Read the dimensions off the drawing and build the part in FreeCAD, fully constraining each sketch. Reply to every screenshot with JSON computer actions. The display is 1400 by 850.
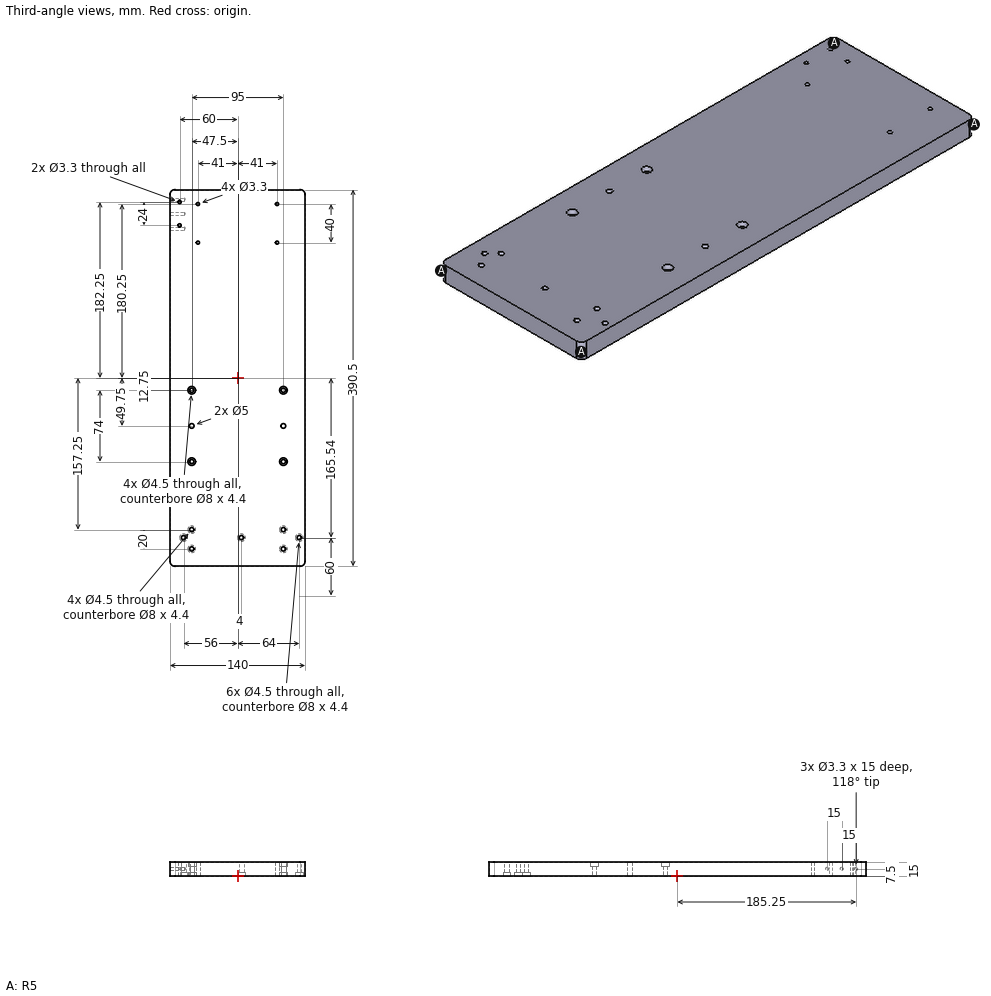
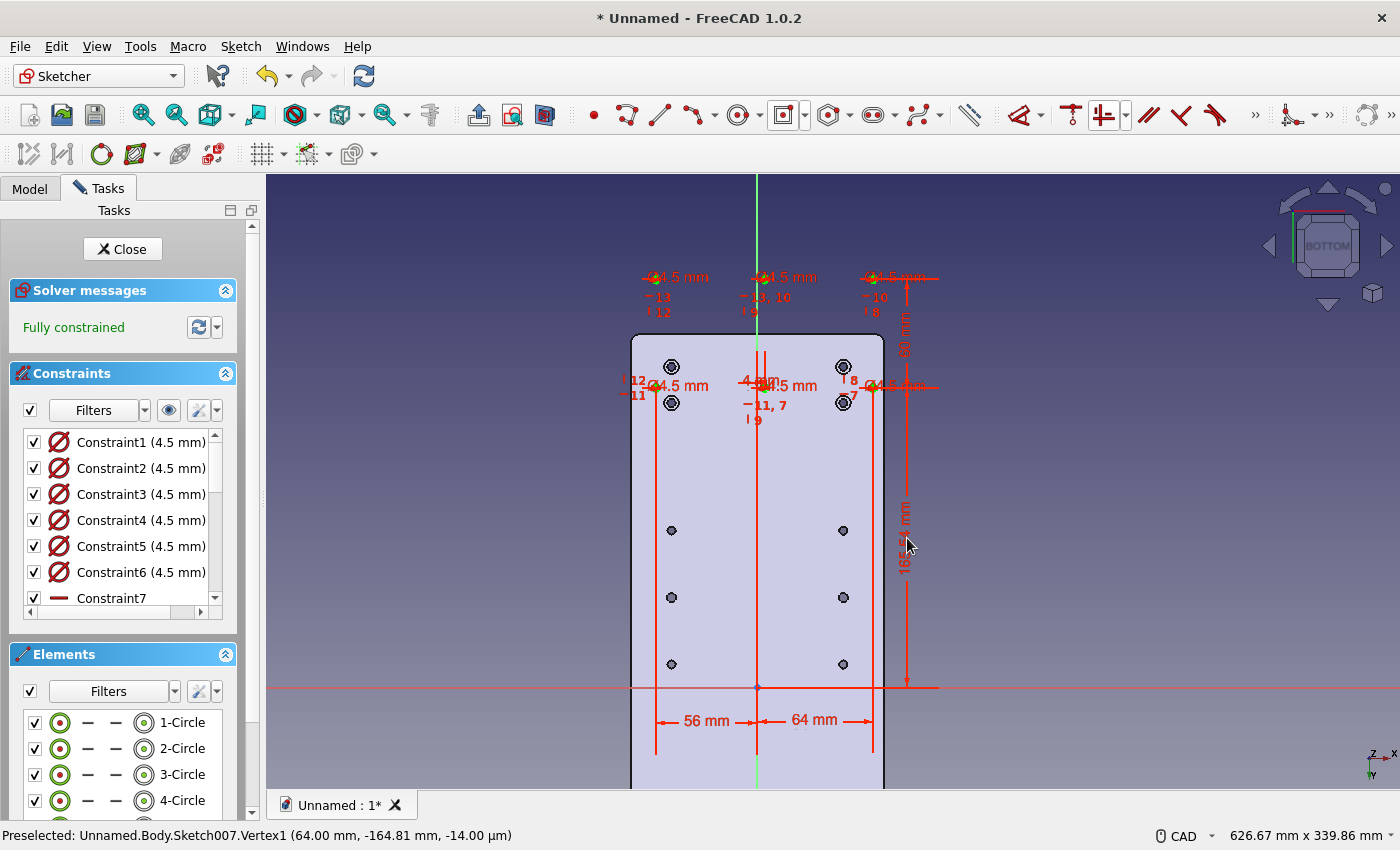
{"action": "left_click", "coordinate": [123, 249]}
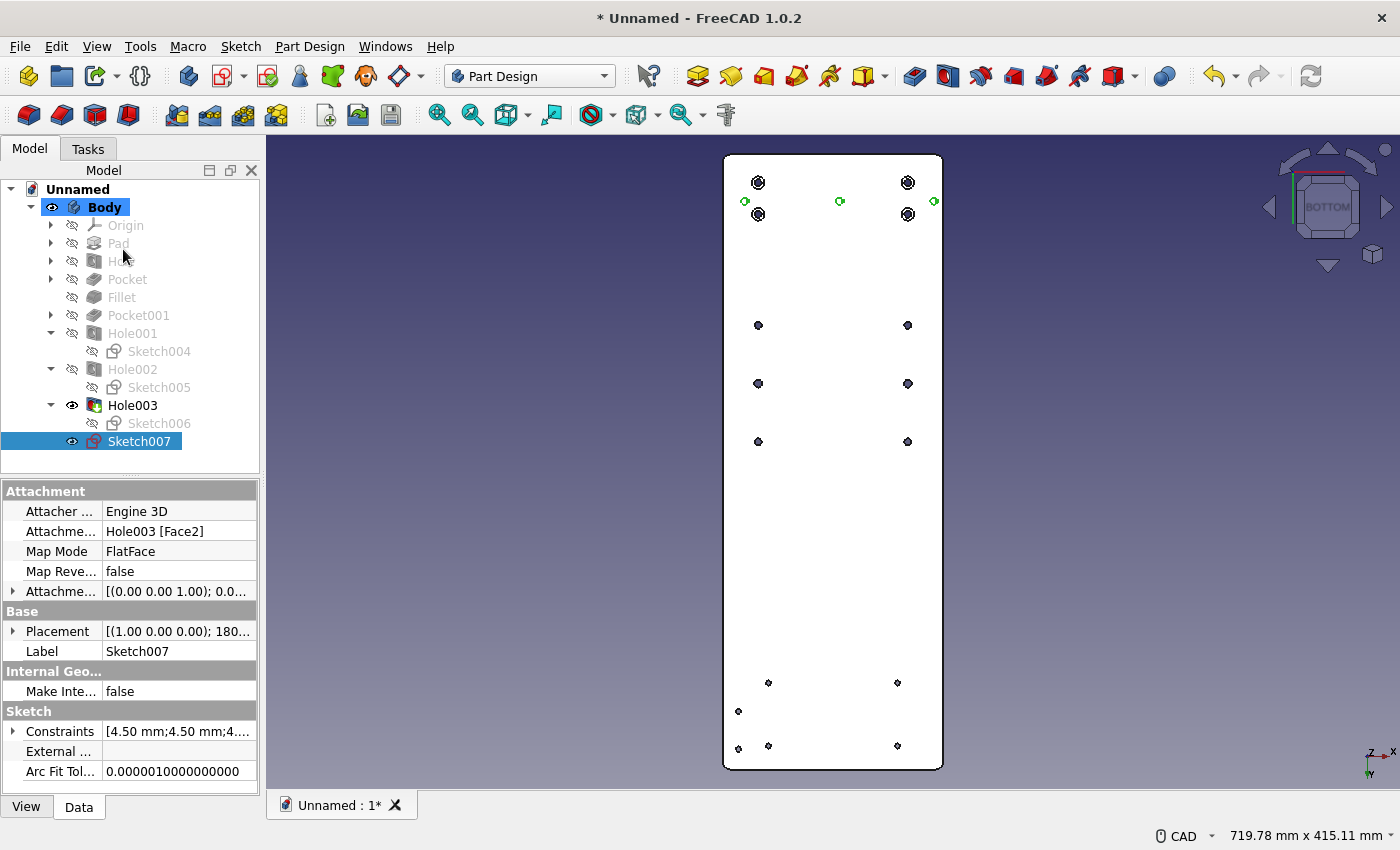
{"action": "left_click", "coordinate": [948, 76]}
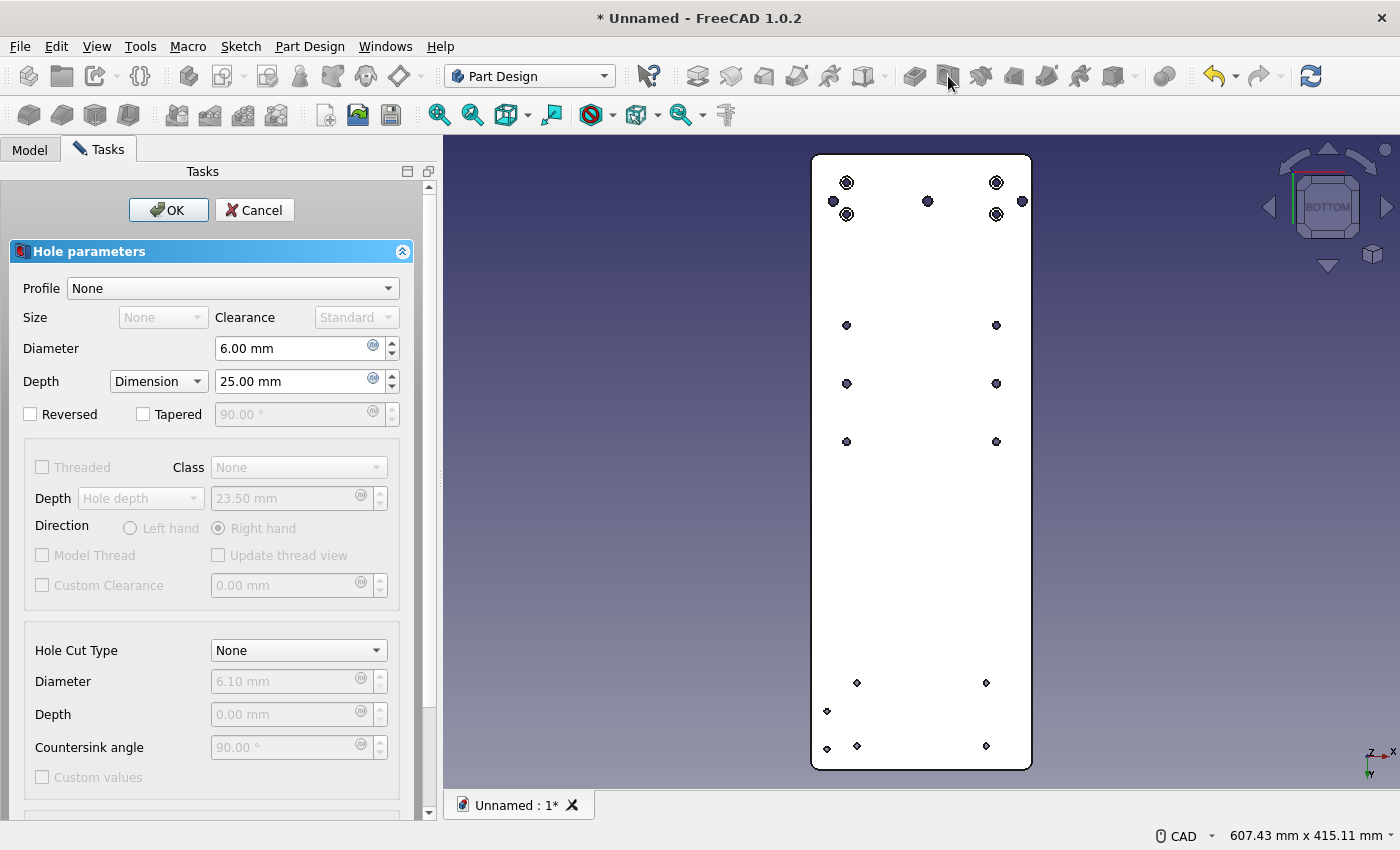
{"action": "triple_click", "coordinate": [300, 348]}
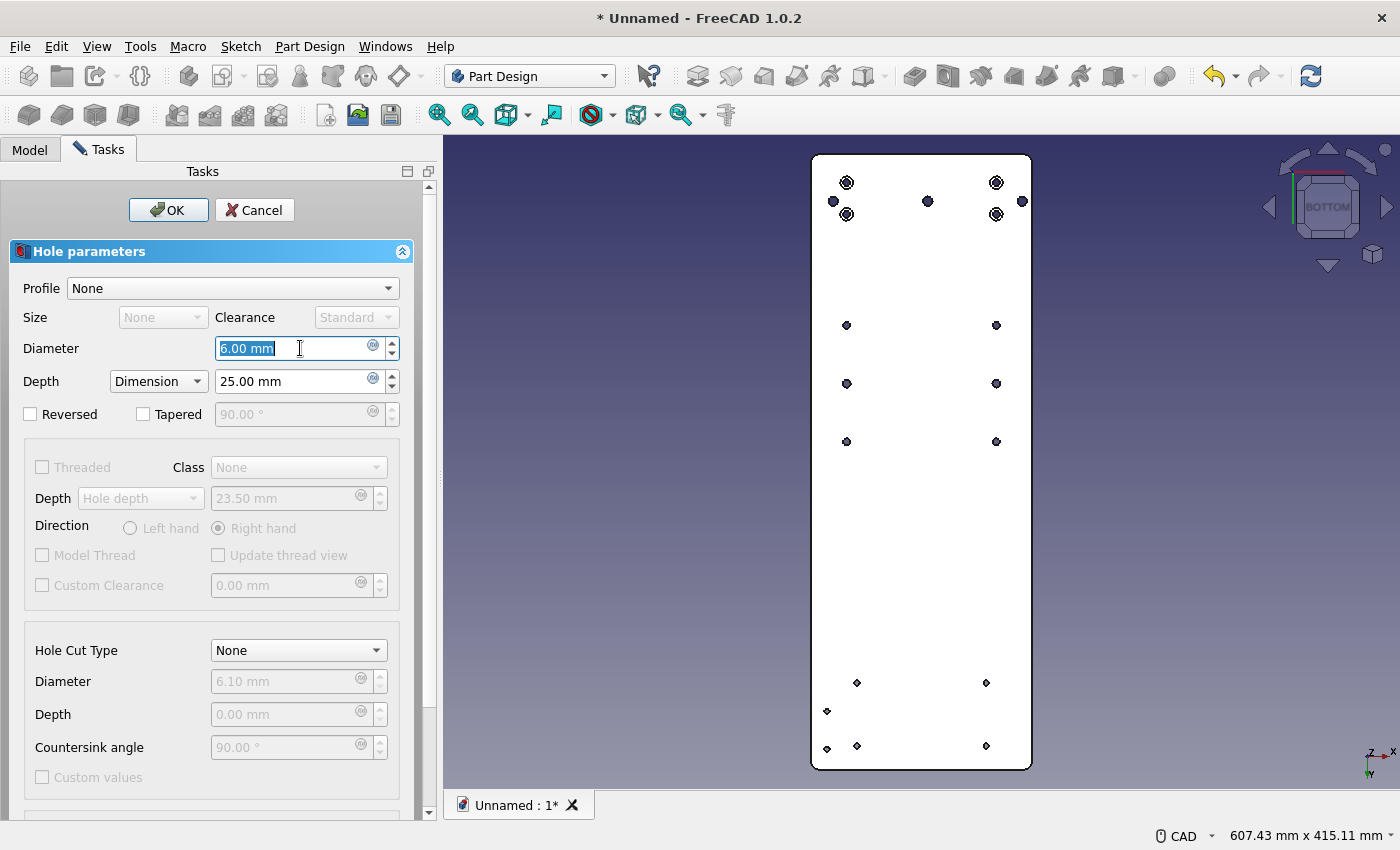
{"action": "type", "text": "4.5"}
{"action": "key", "text": "Tab"}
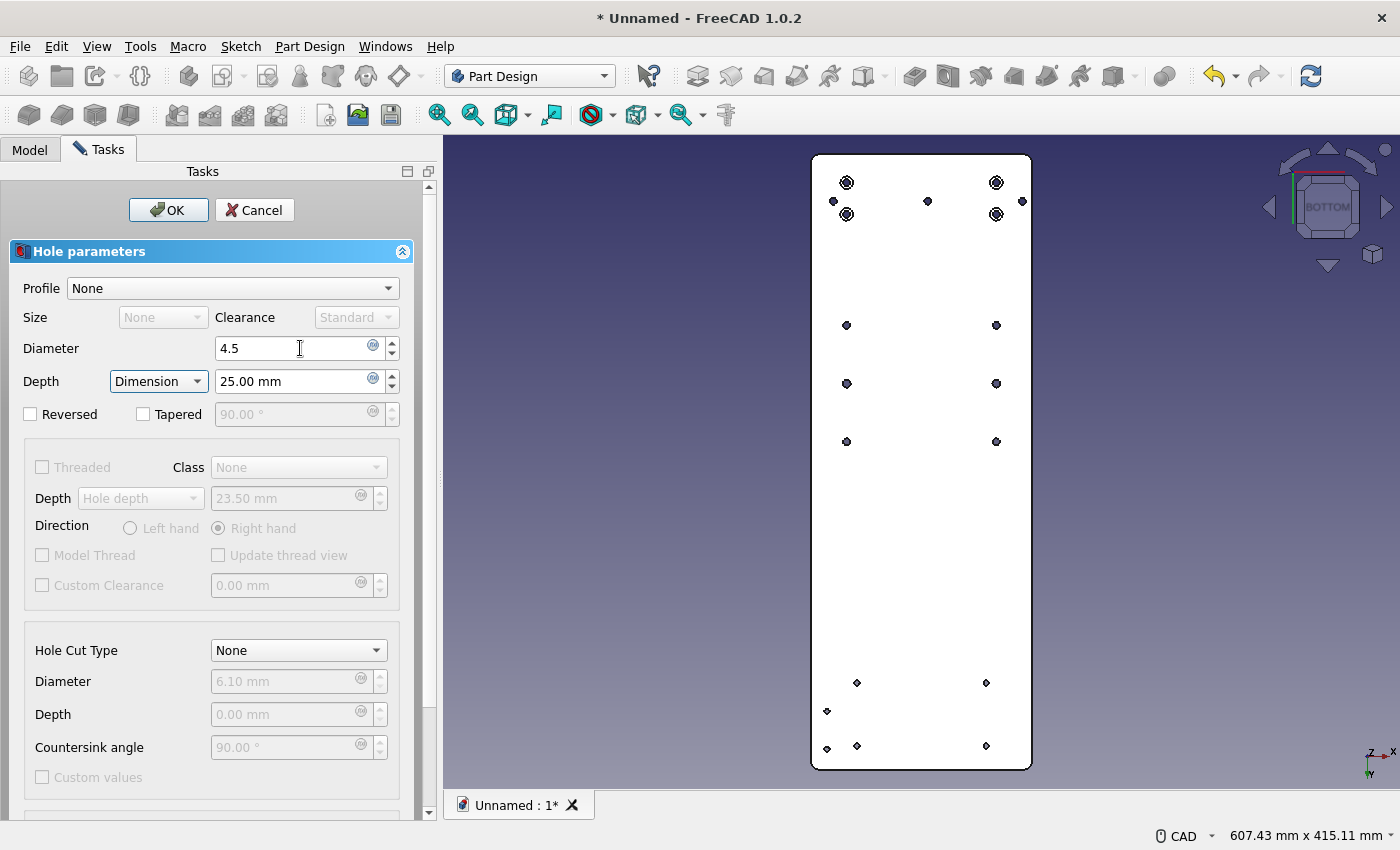
{"action": "left_click", "coordinate": [160, 382]}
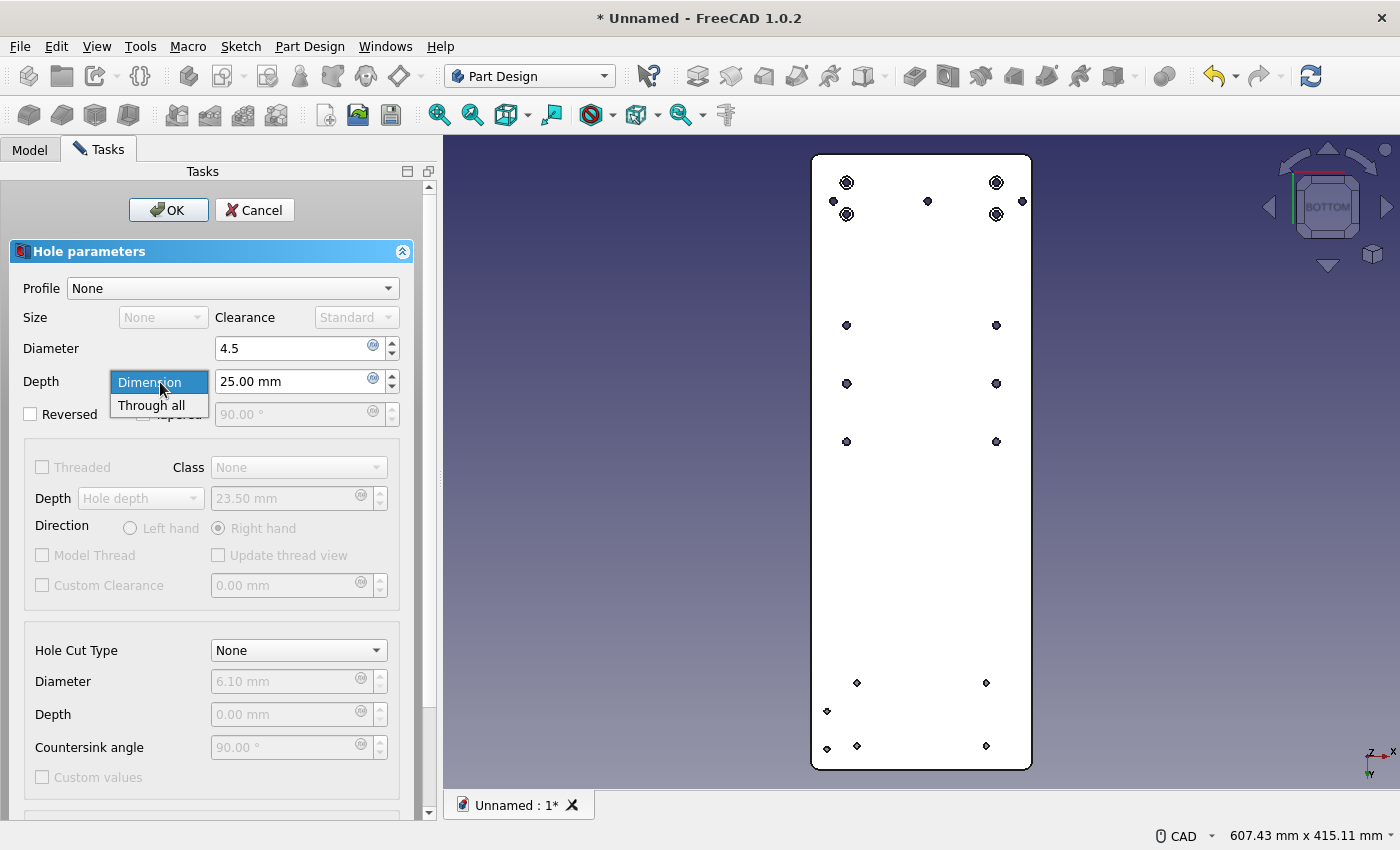
{"action": "left_click", "coordinate": [158, 406]}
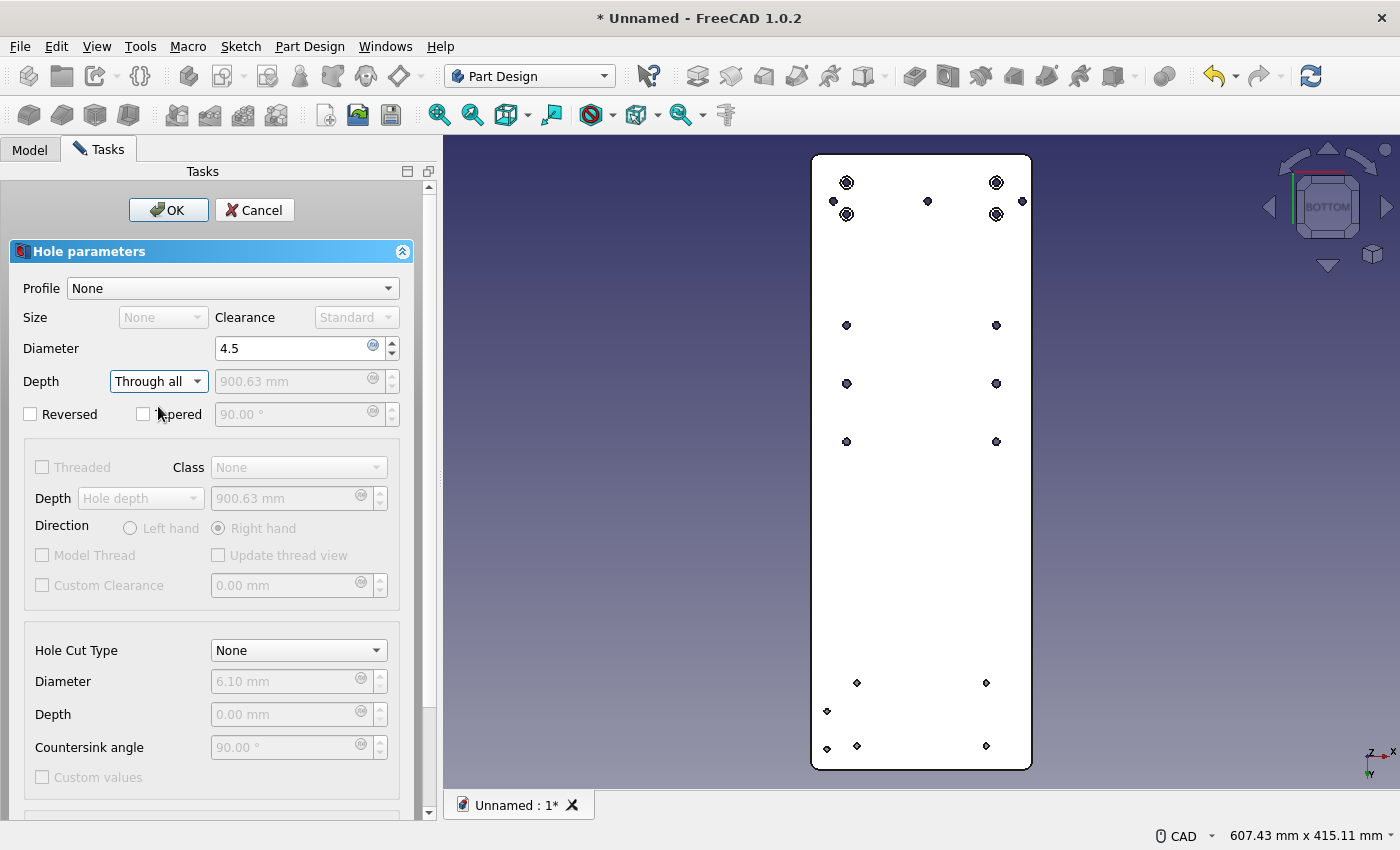
{"action": "left_click", "coordinate": [300, 650]}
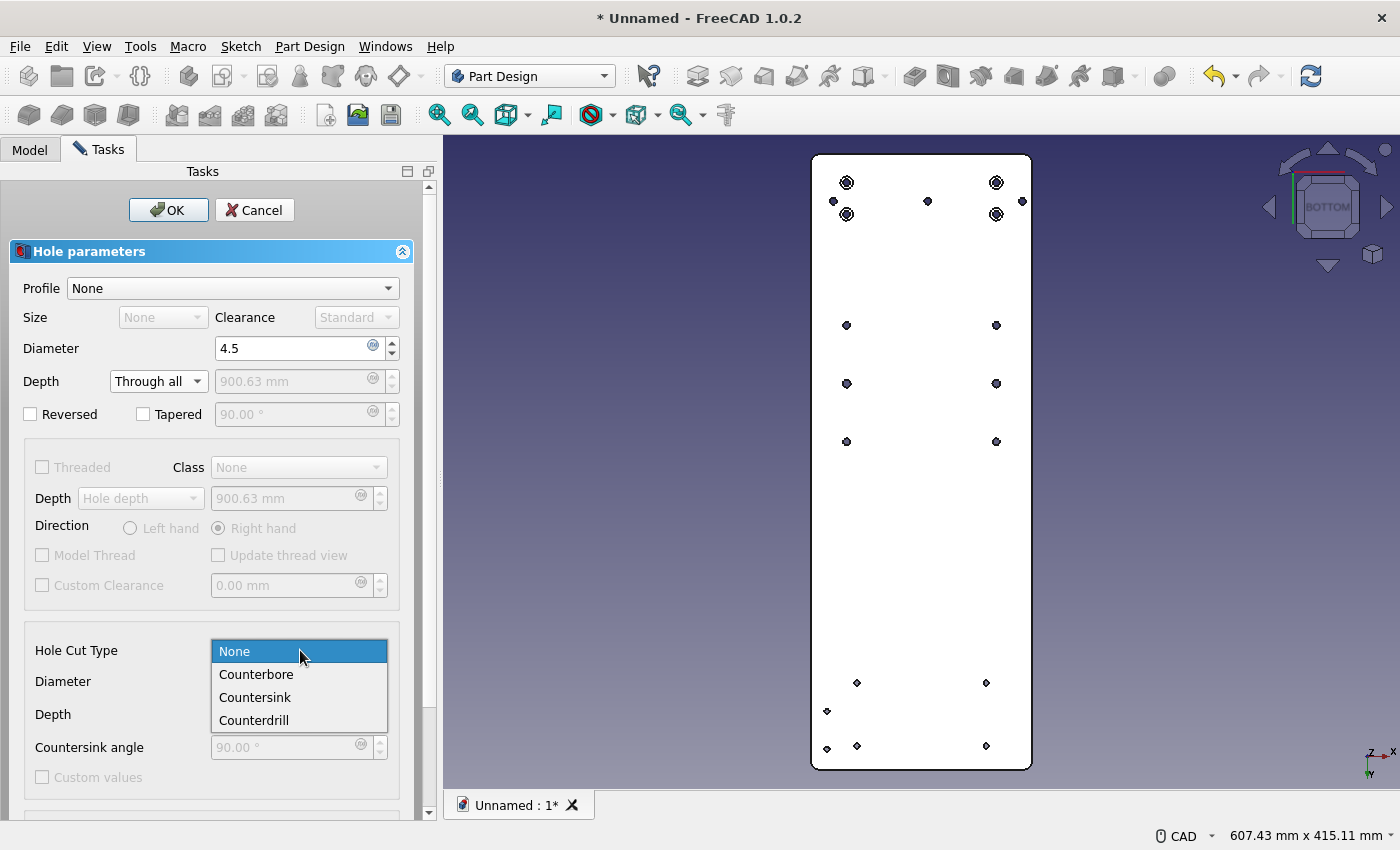
{"action": "left_click", "coordinate": [298, 674]}